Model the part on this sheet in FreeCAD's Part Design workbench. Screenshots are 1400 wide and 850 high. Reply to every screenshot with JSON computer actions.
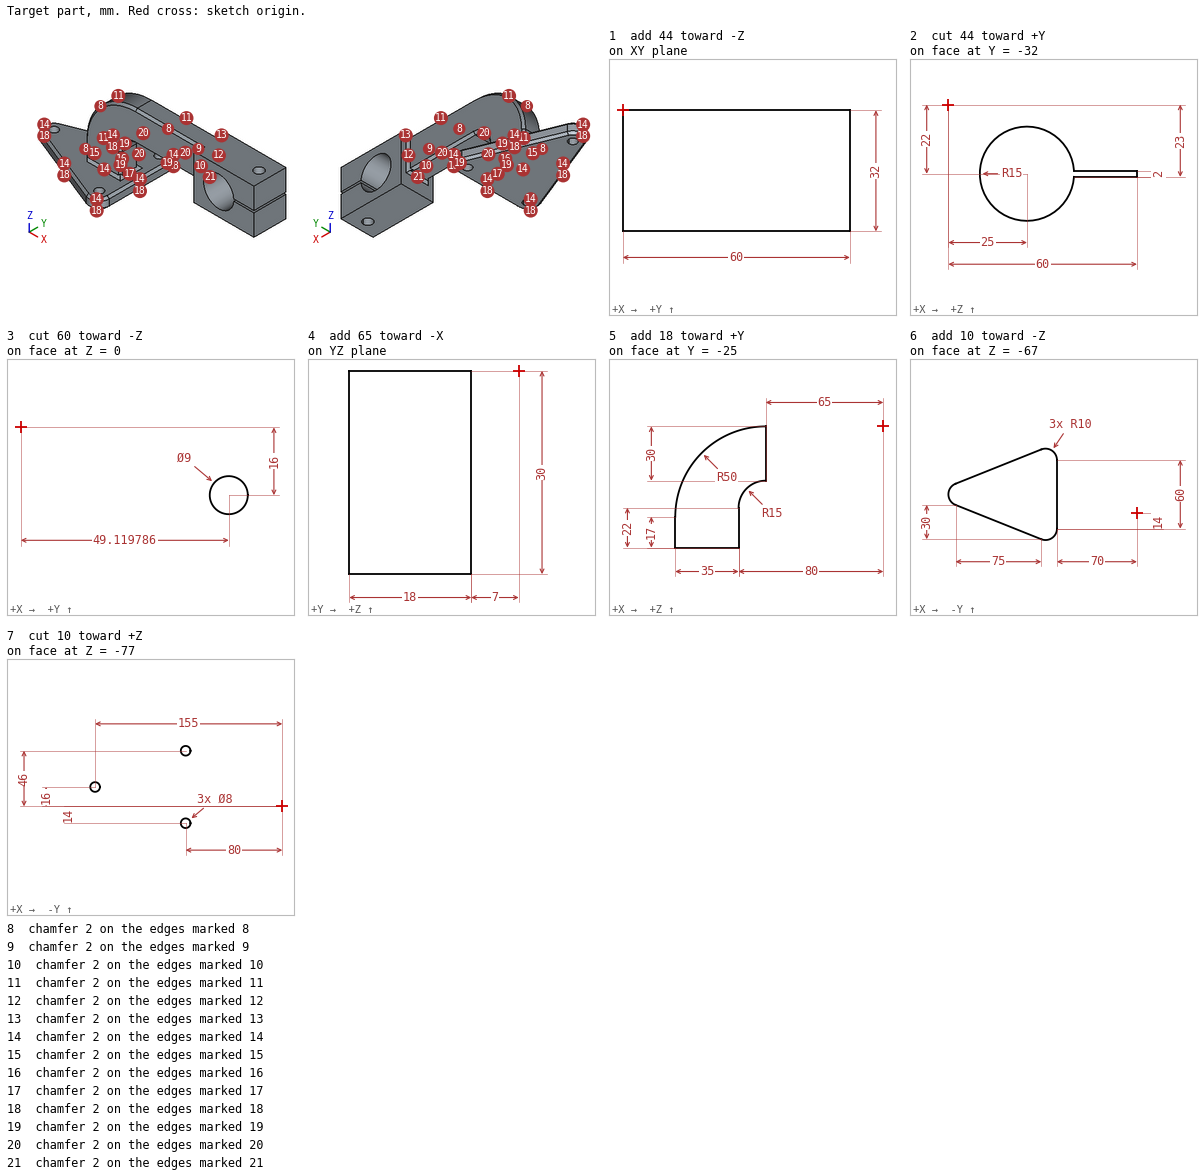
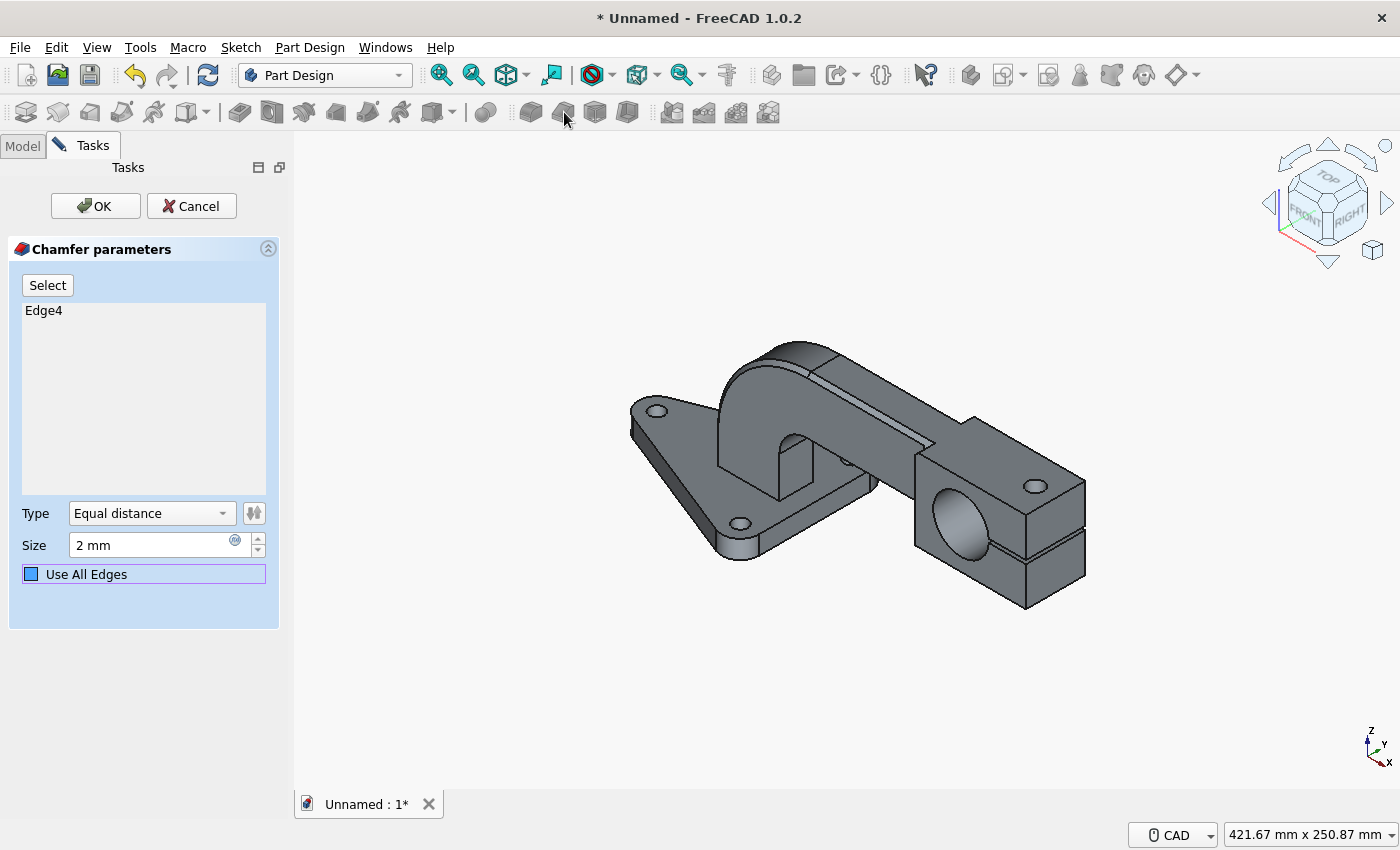
{"action": "left_click", "coordinate": [96, 206]}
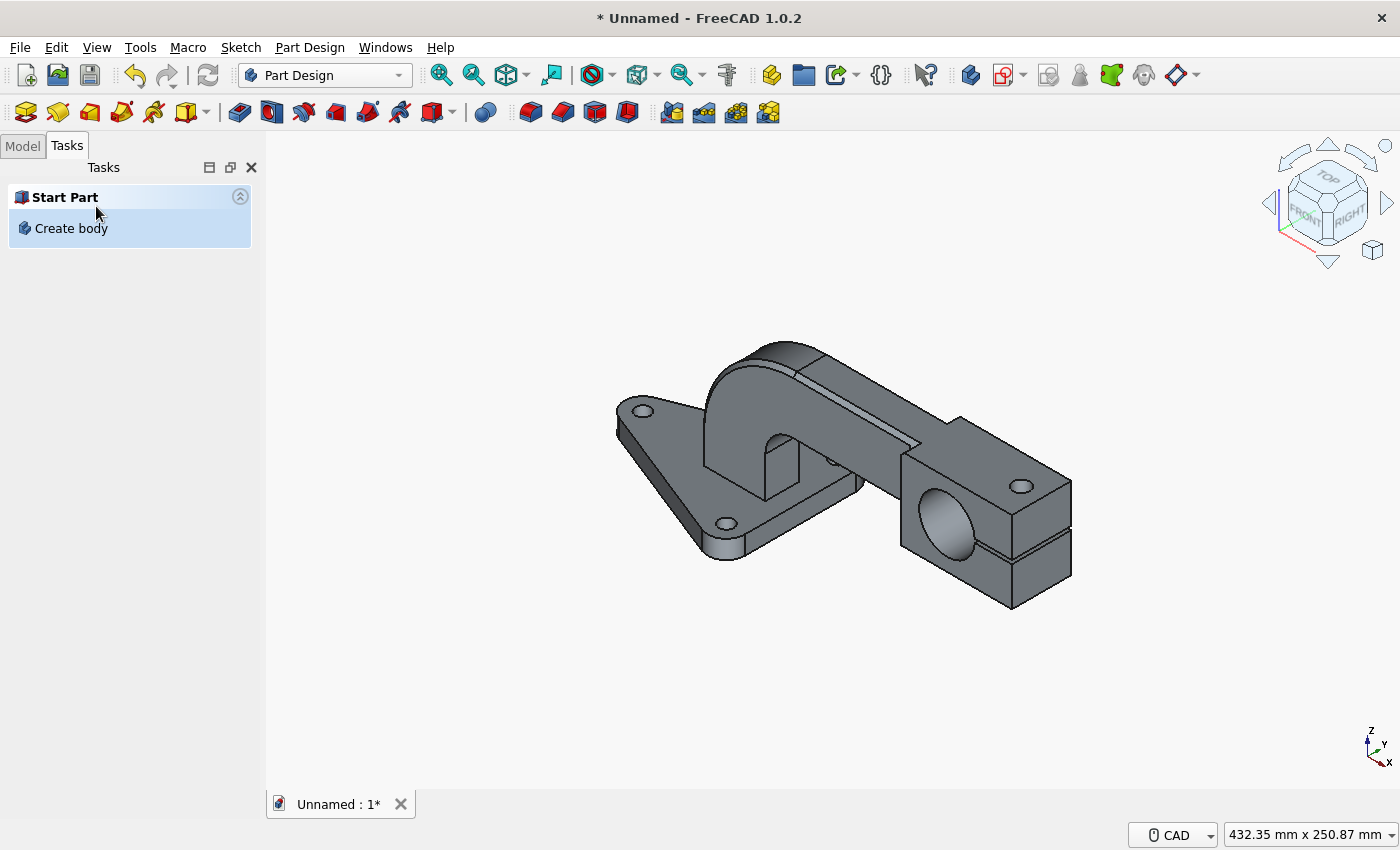
{"action": "key", "text": "2"}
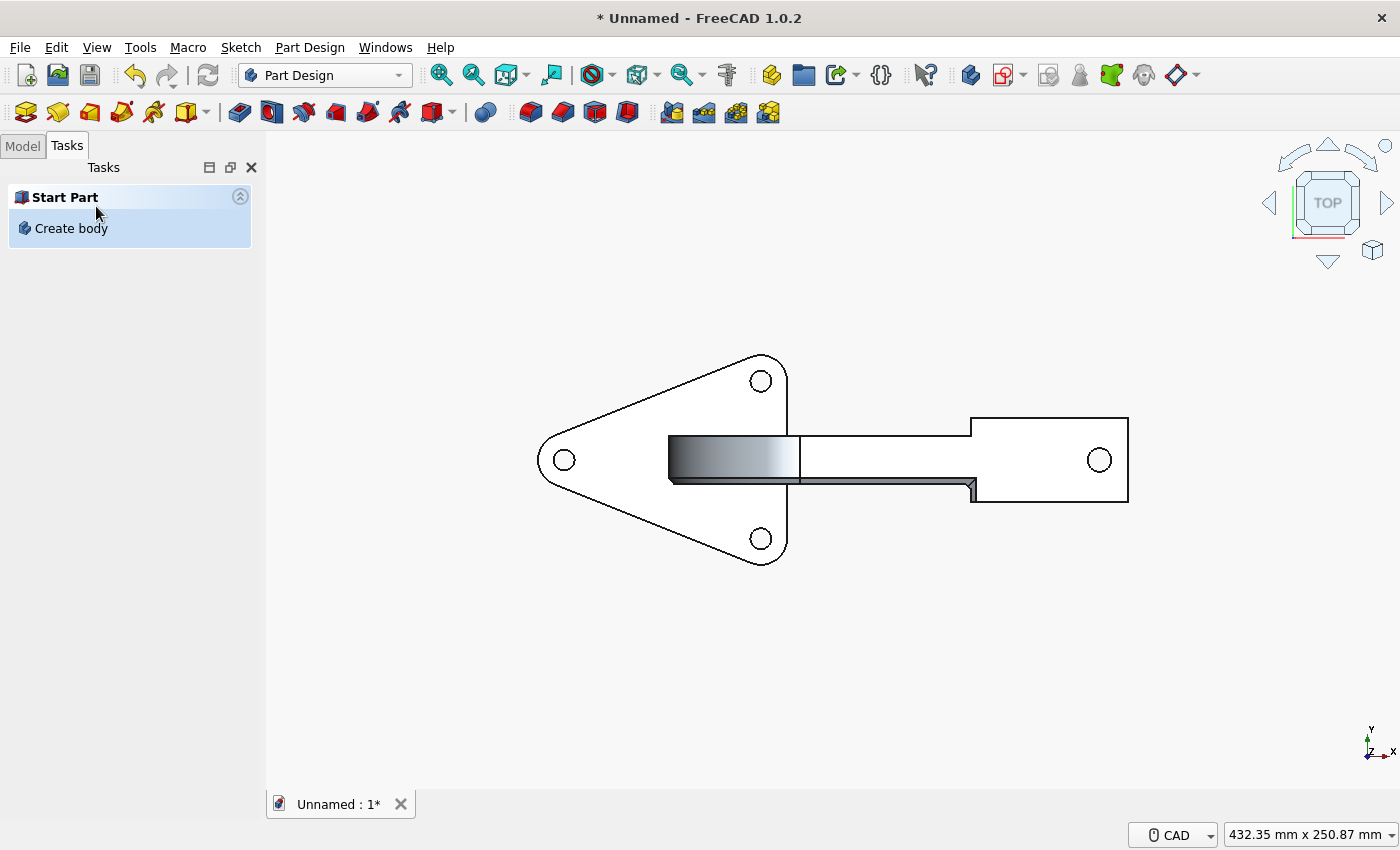
{"action": "left_click", "coordinate": [707, 435]}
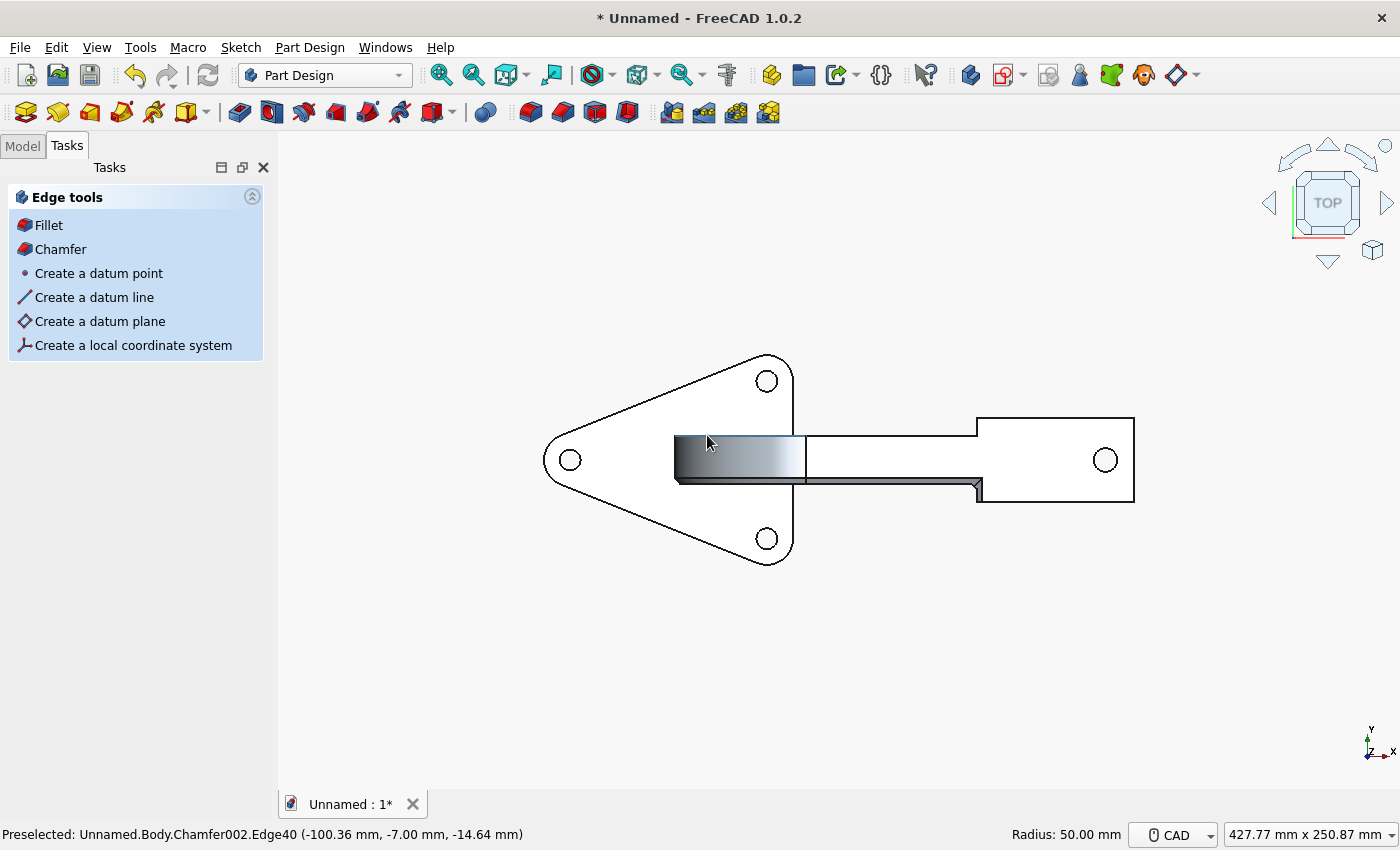
{"action": "key", "text": "0"}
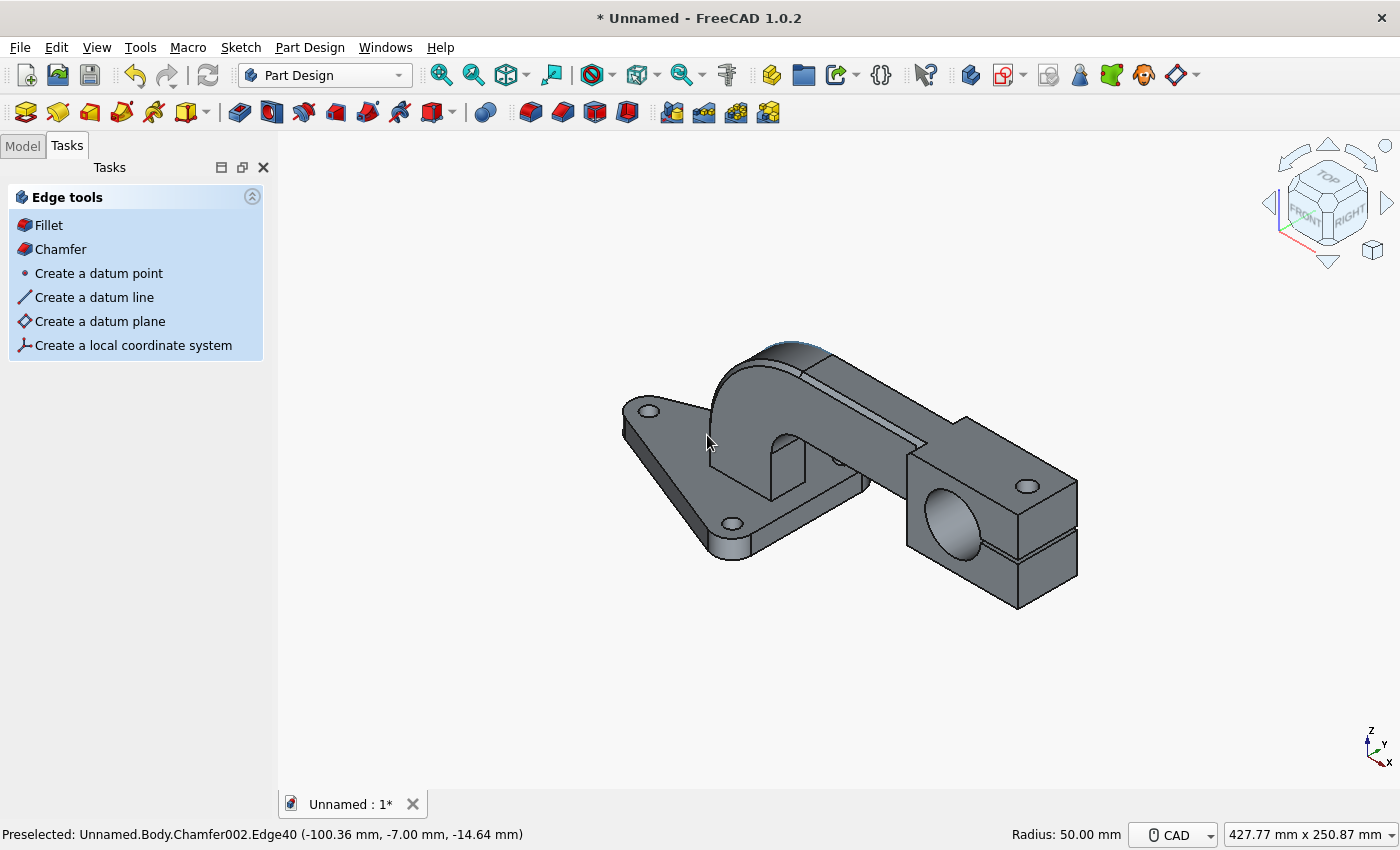
{"action": "key", "text": "1"}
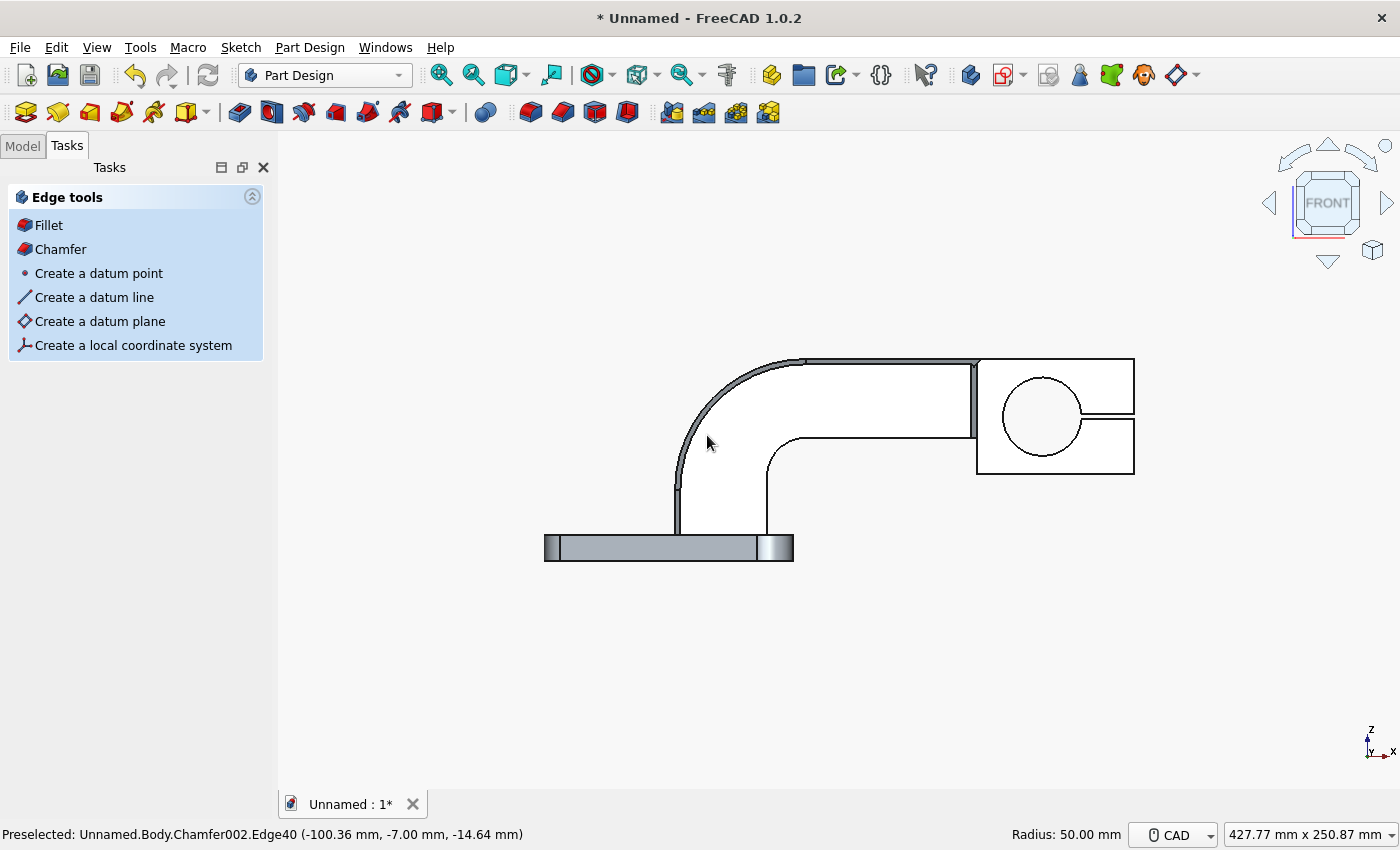
{"action": "key", "text": "3"}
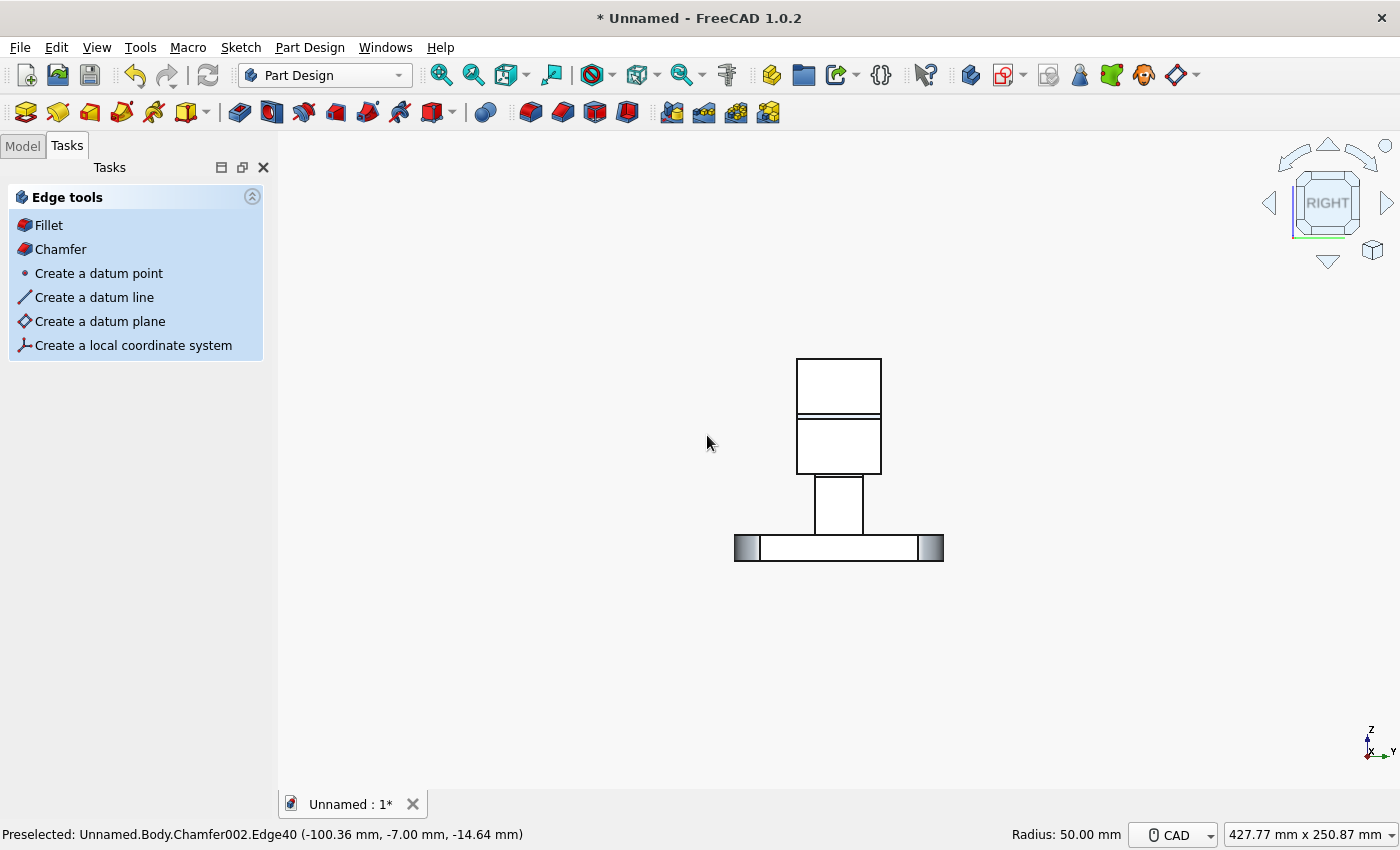
{"action": "key", "text": "v f"}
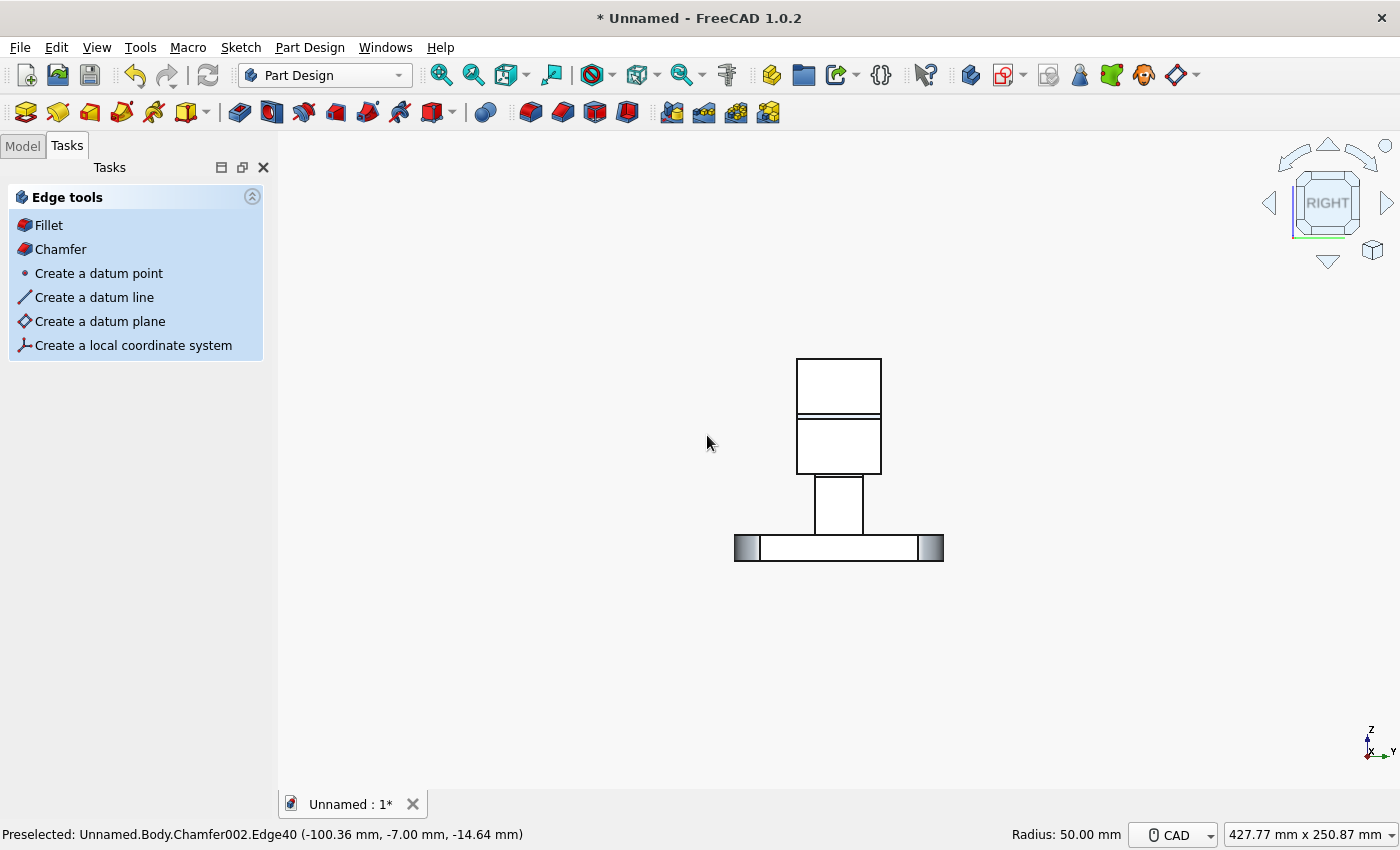
{"action": "key", "text": "5"}